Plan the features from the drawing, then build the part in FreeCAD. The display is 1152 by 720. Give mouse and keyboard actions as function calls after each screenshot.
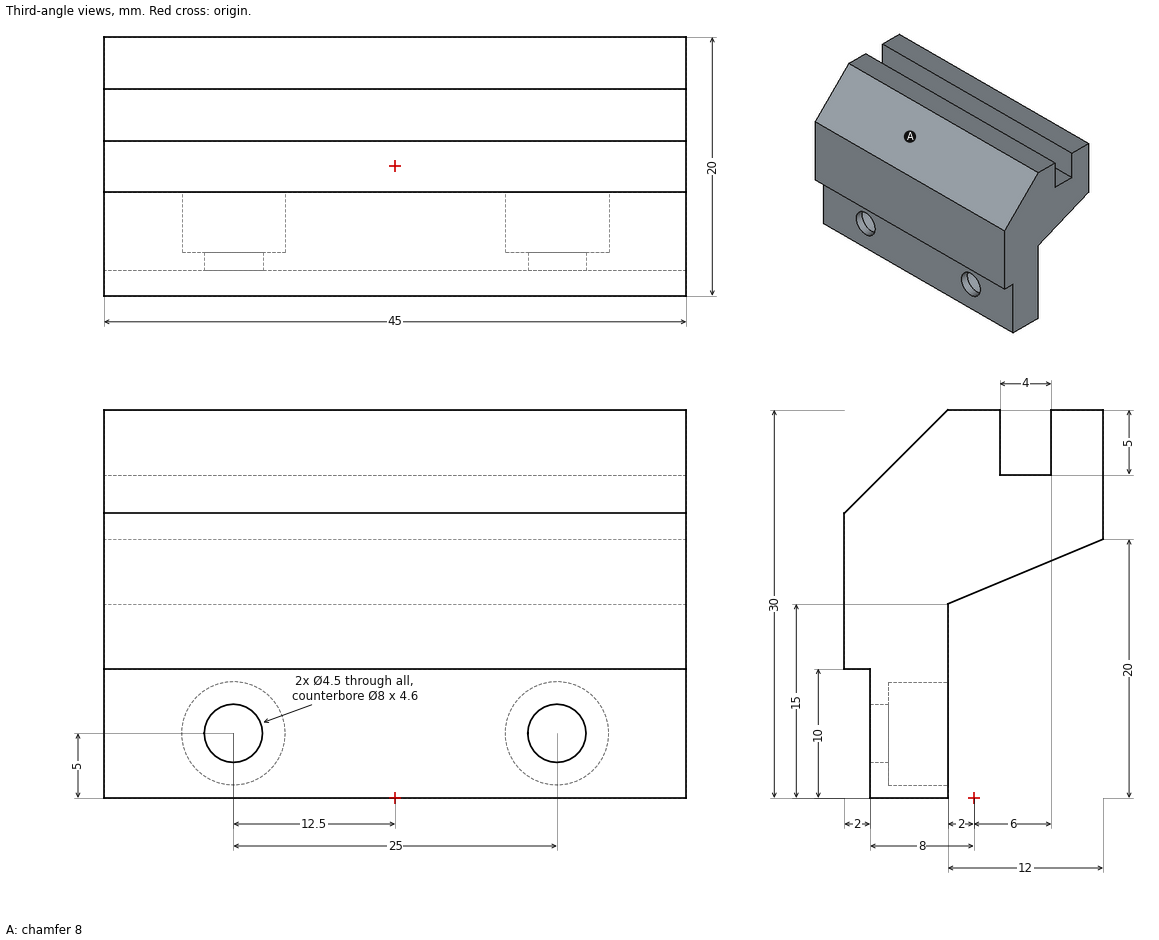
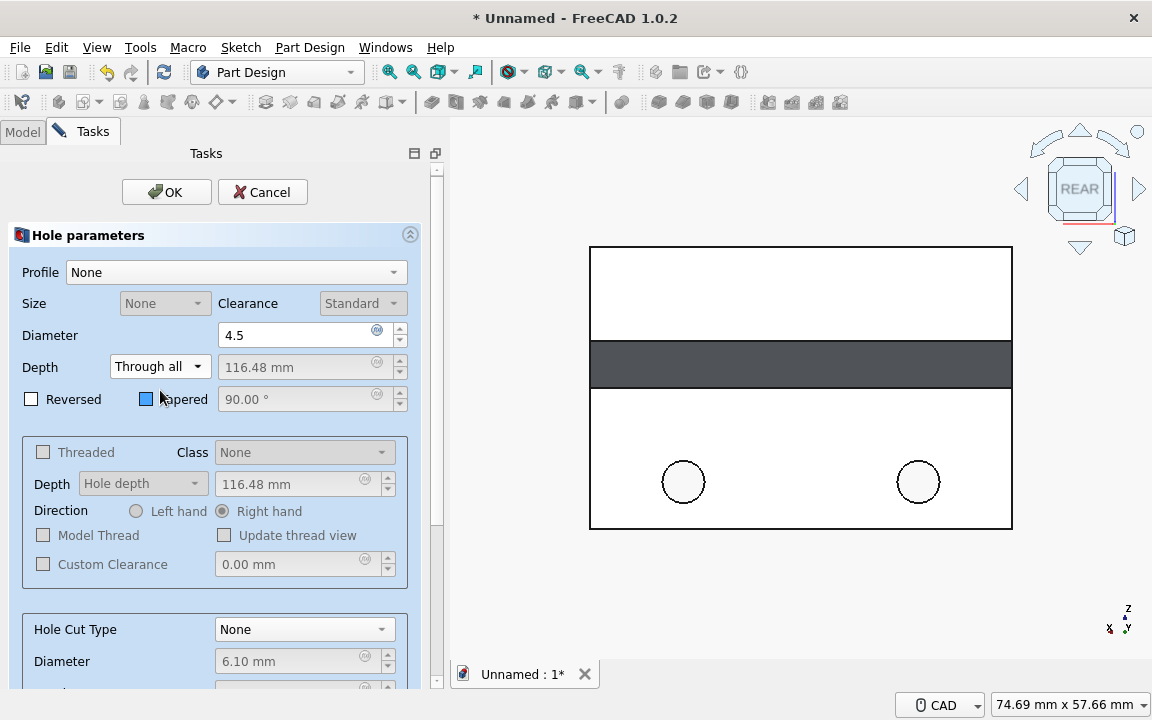
click(306, 630)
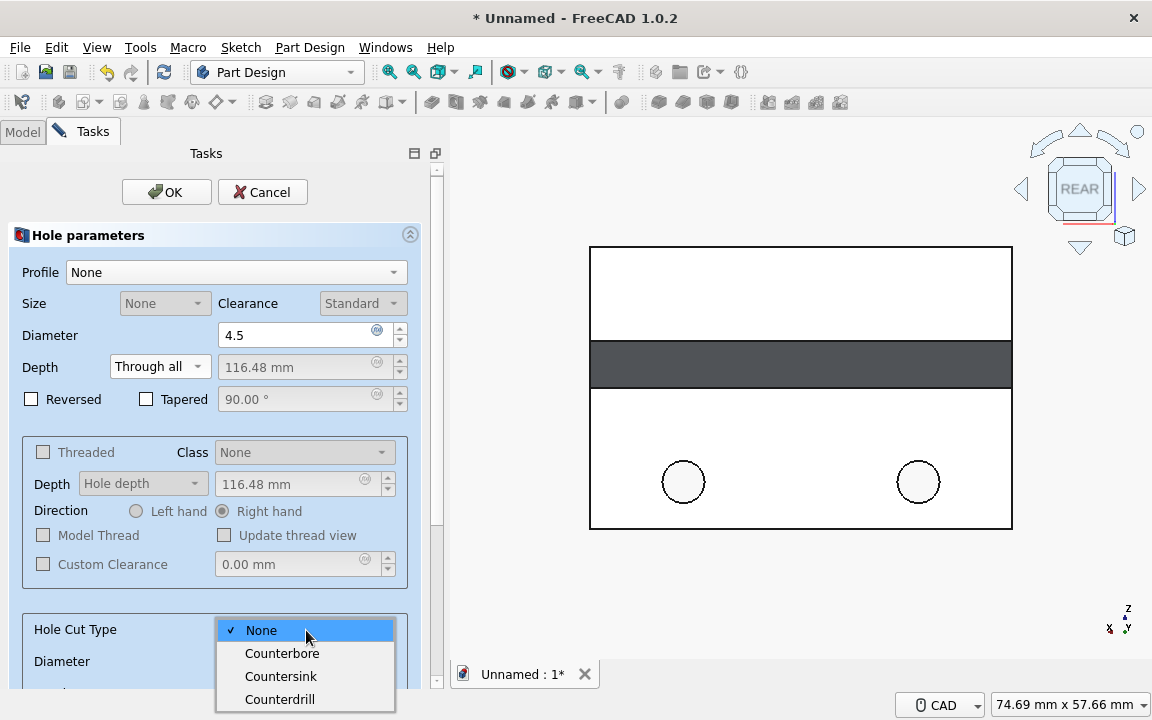
click(304, 654)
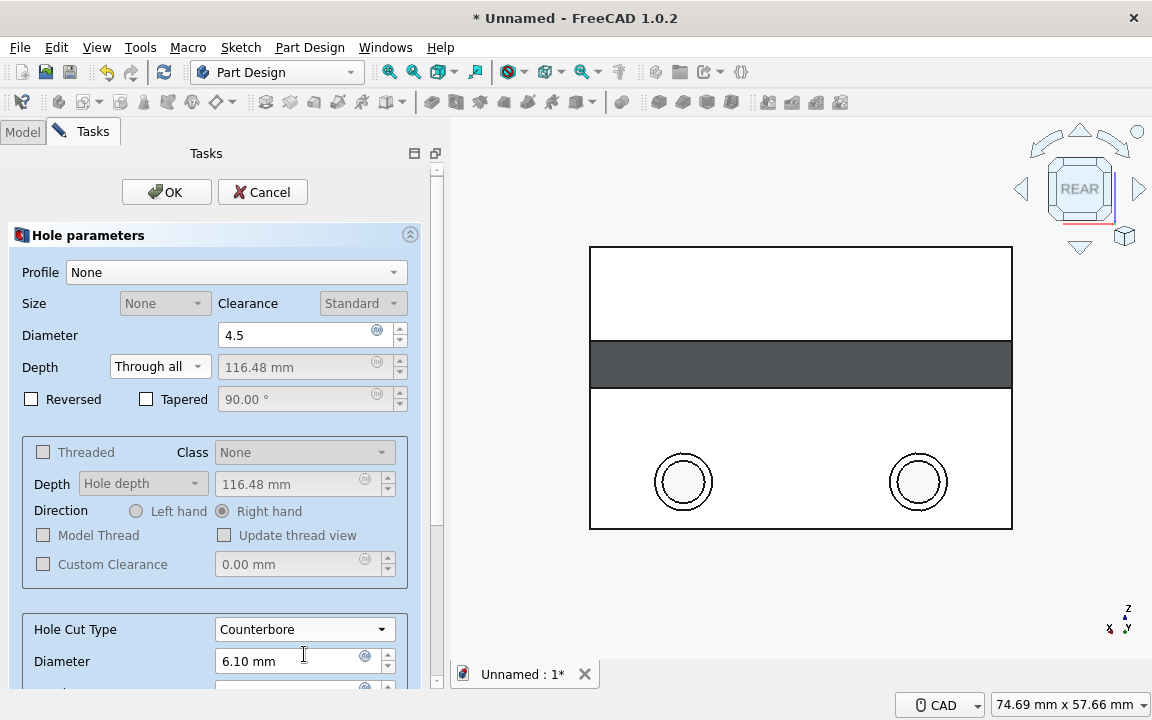
triple_click(298, 661)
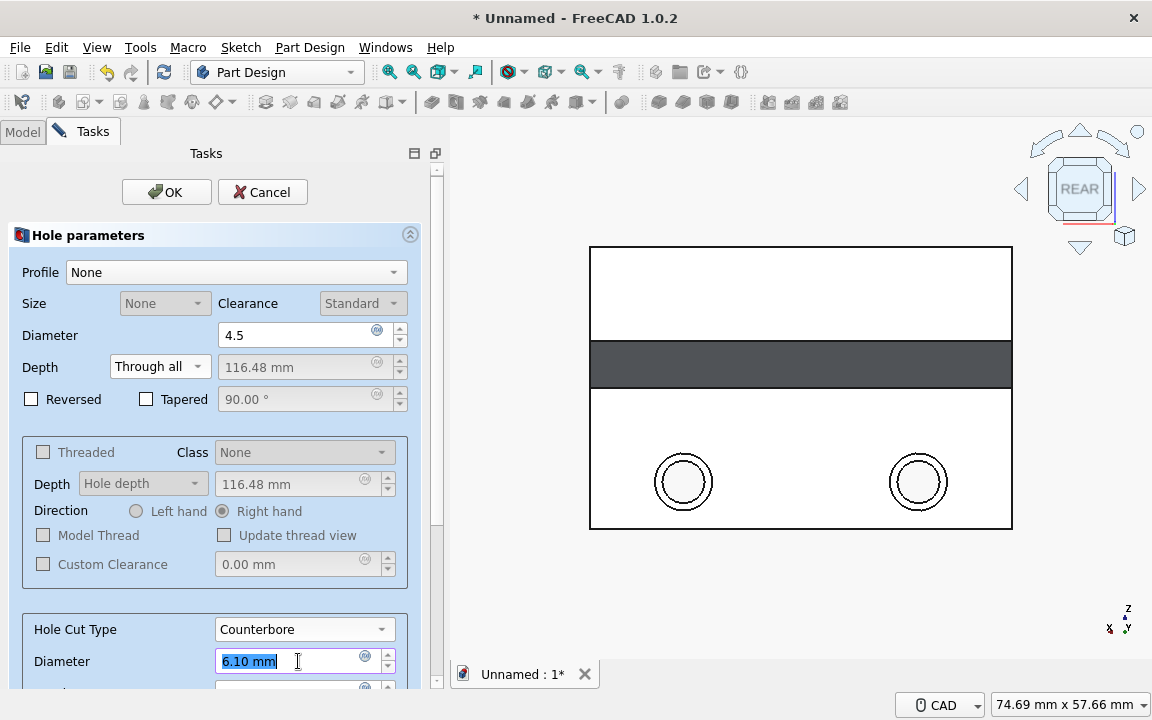
text(8)
key(Tab)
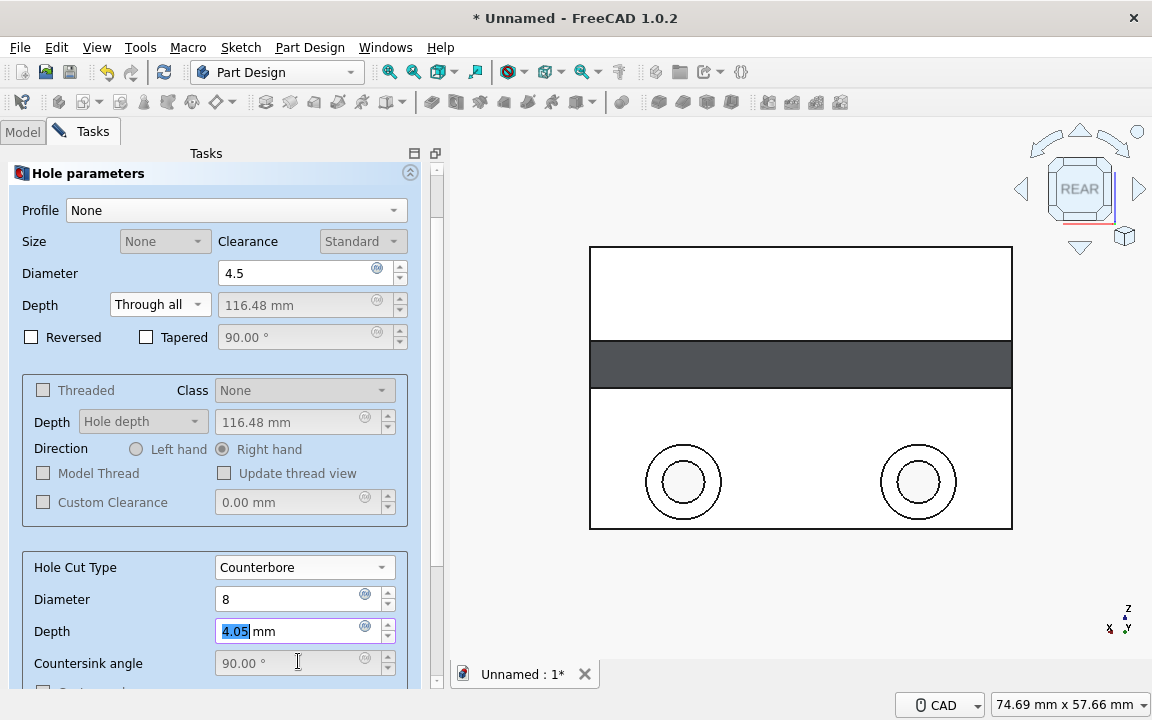
text(4.6)
key(Tab)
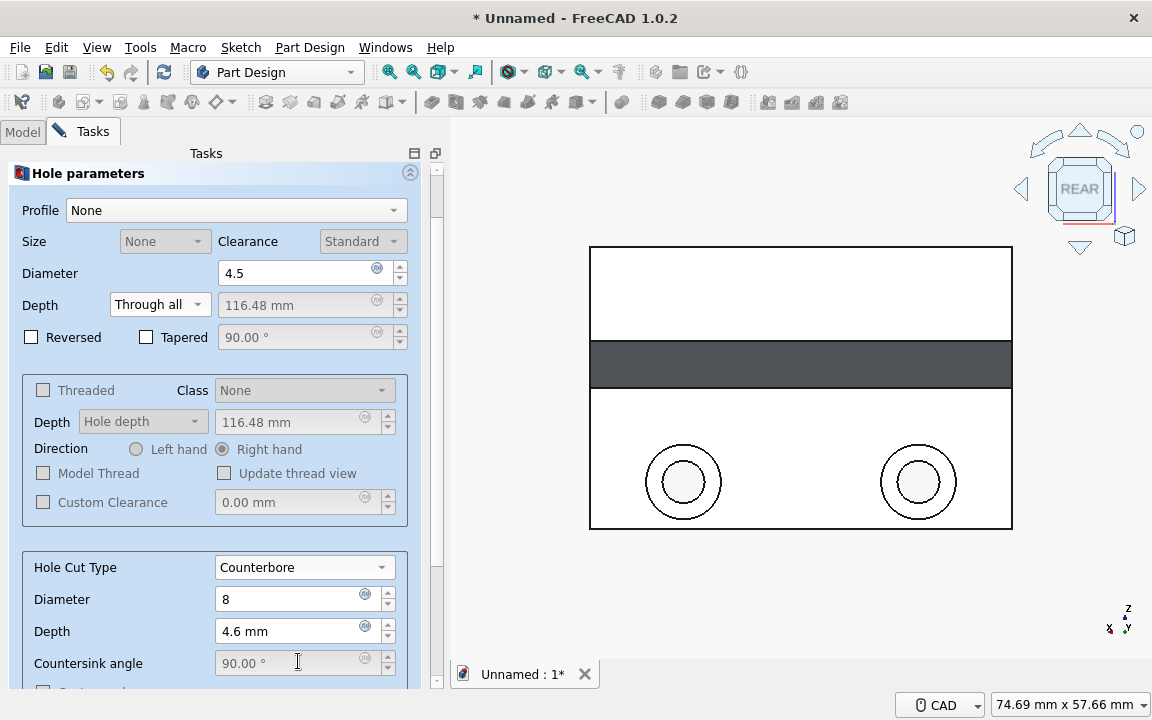
scroll(437, 426, up, 2)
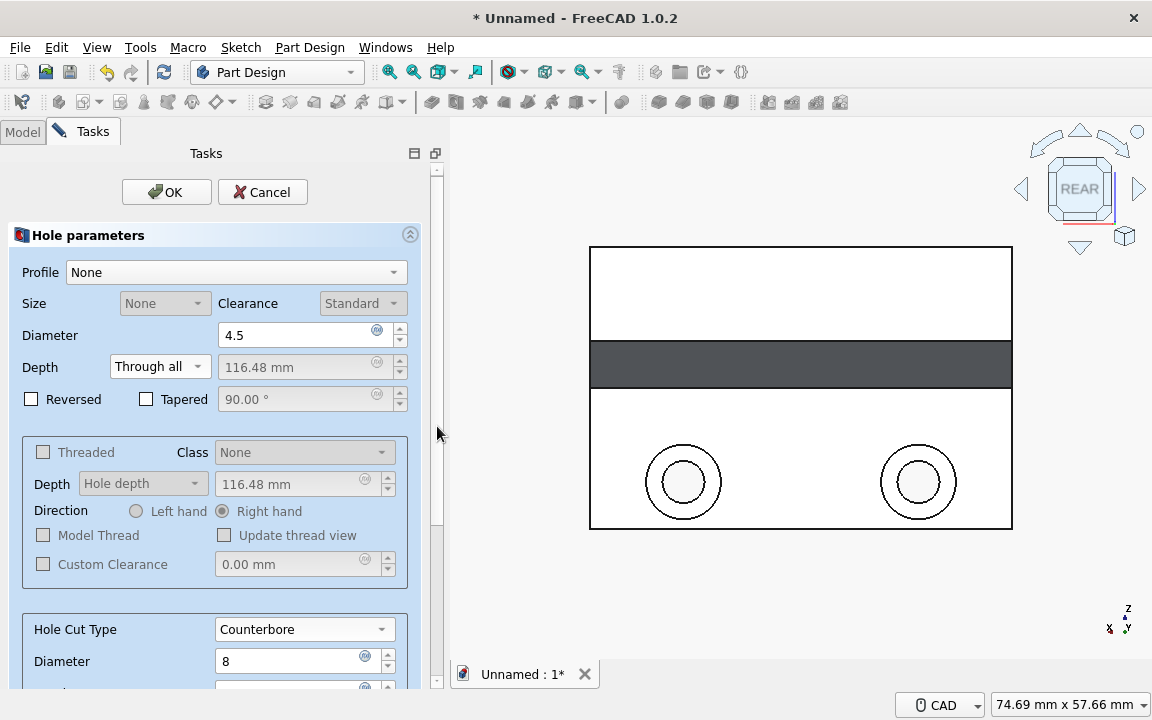
click(167, 192)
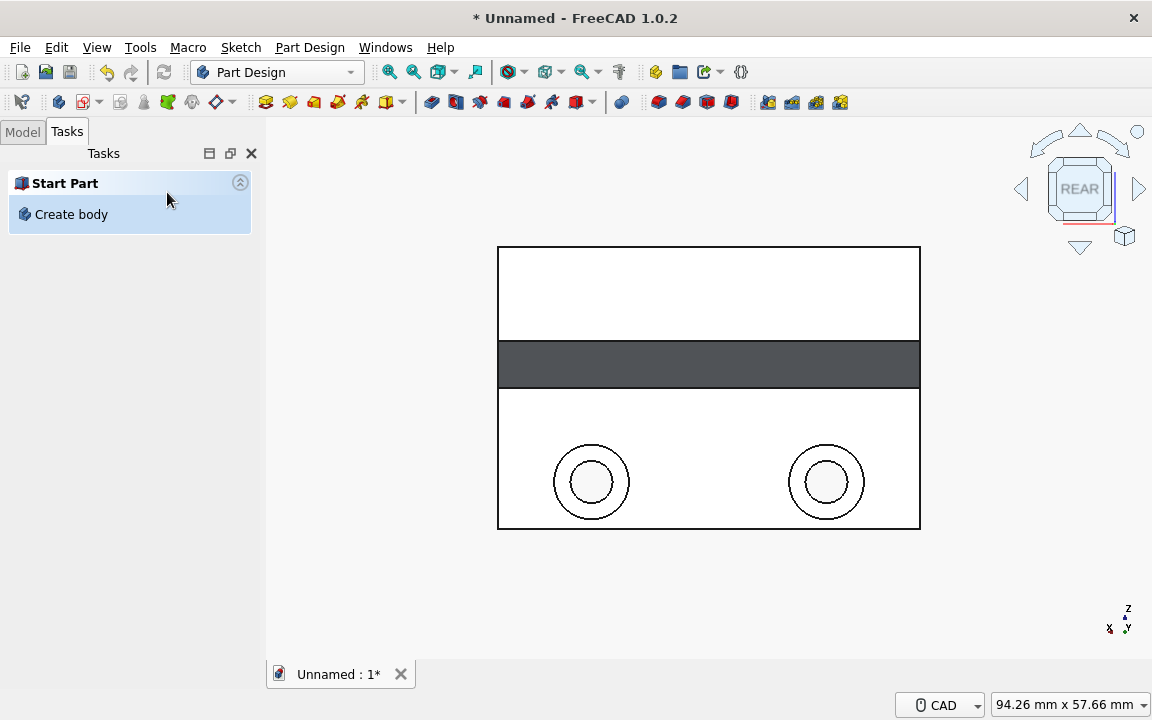
key(6)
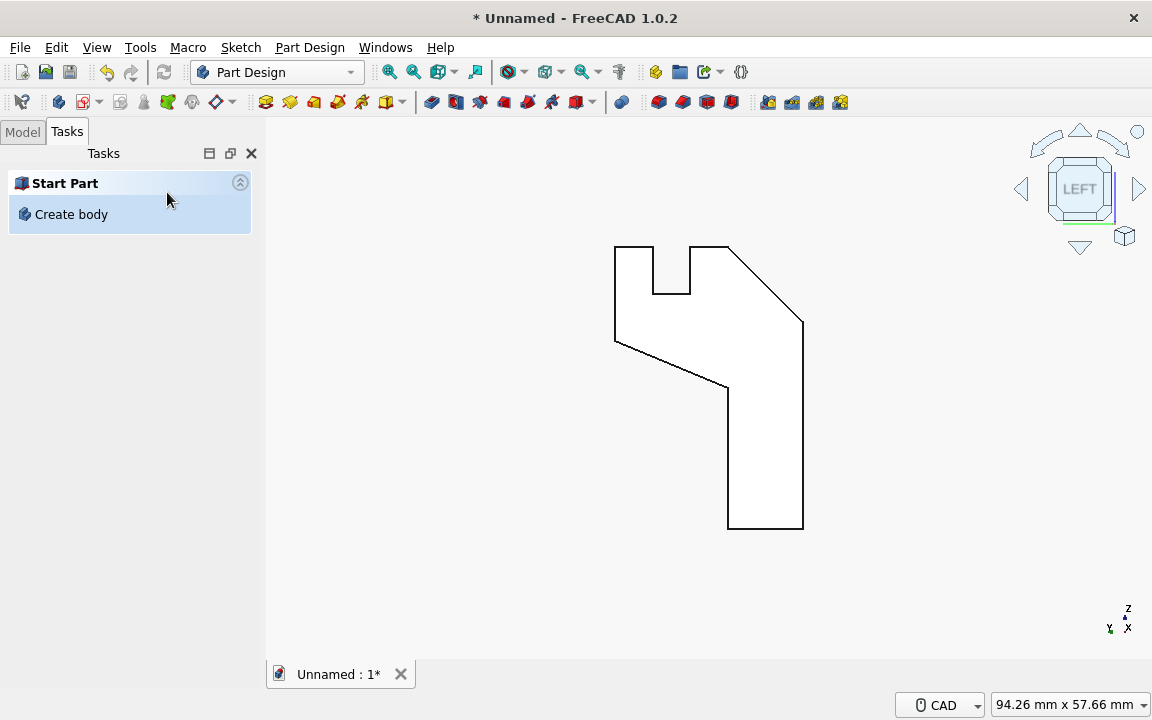
click(763, 347)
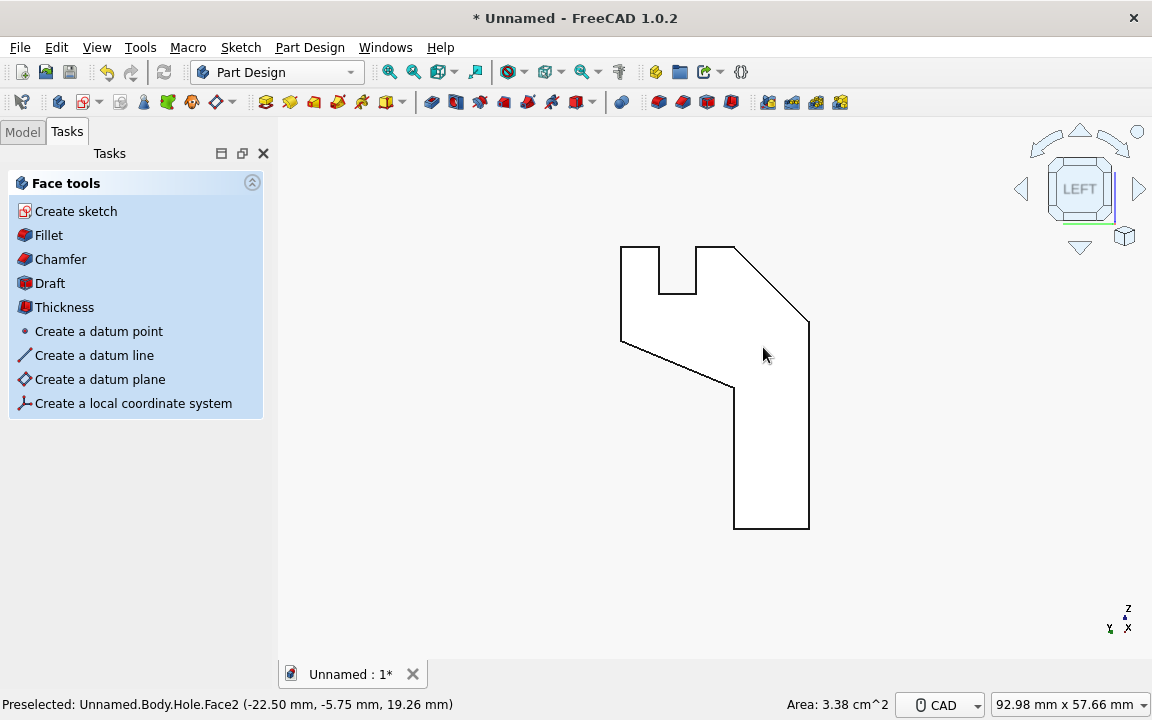
click(84, 102)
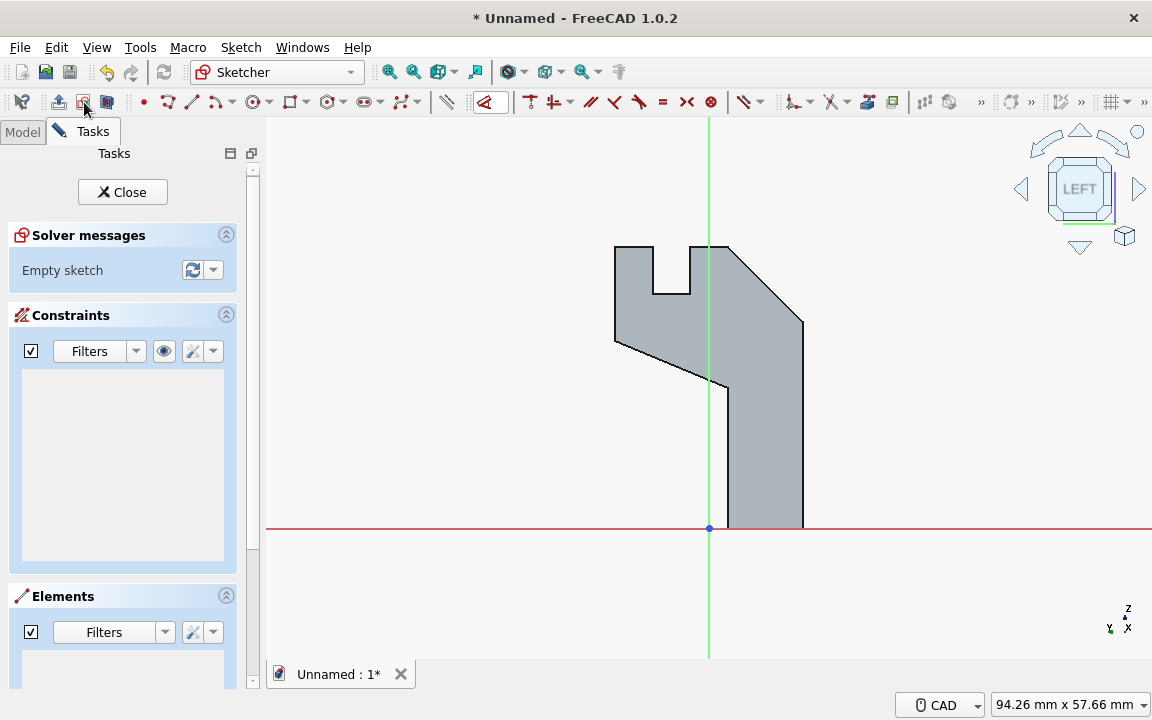
scroll(806, 523, up, 6)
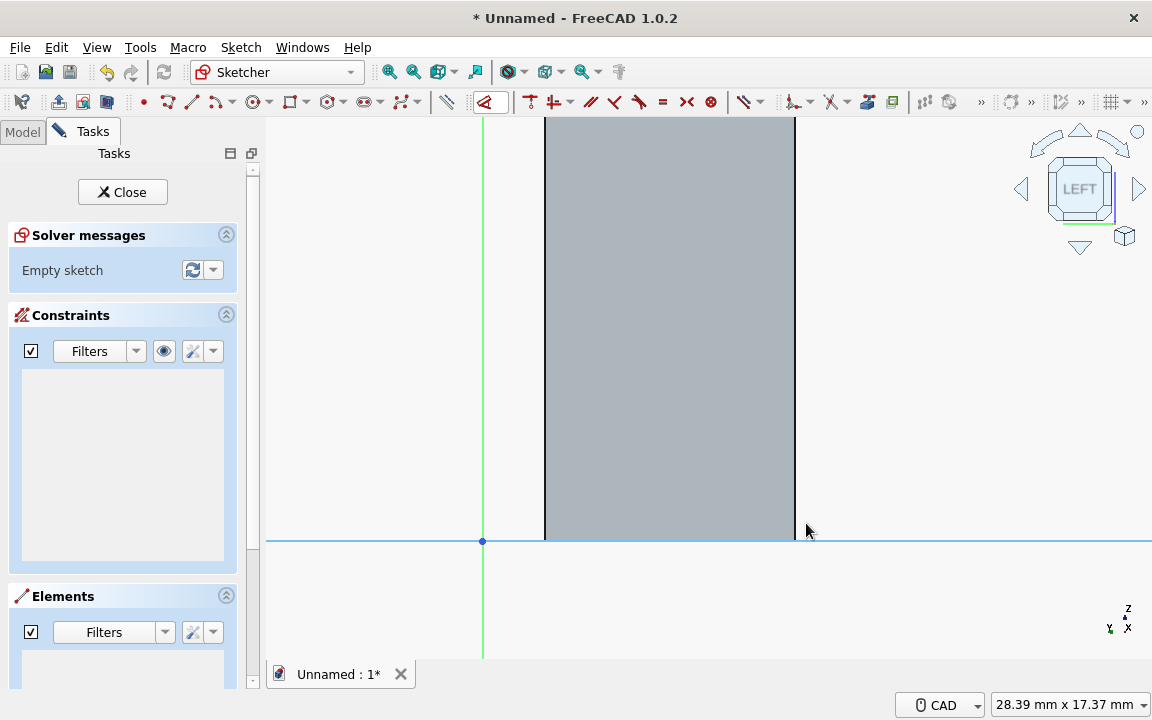
key(g)
key(r)